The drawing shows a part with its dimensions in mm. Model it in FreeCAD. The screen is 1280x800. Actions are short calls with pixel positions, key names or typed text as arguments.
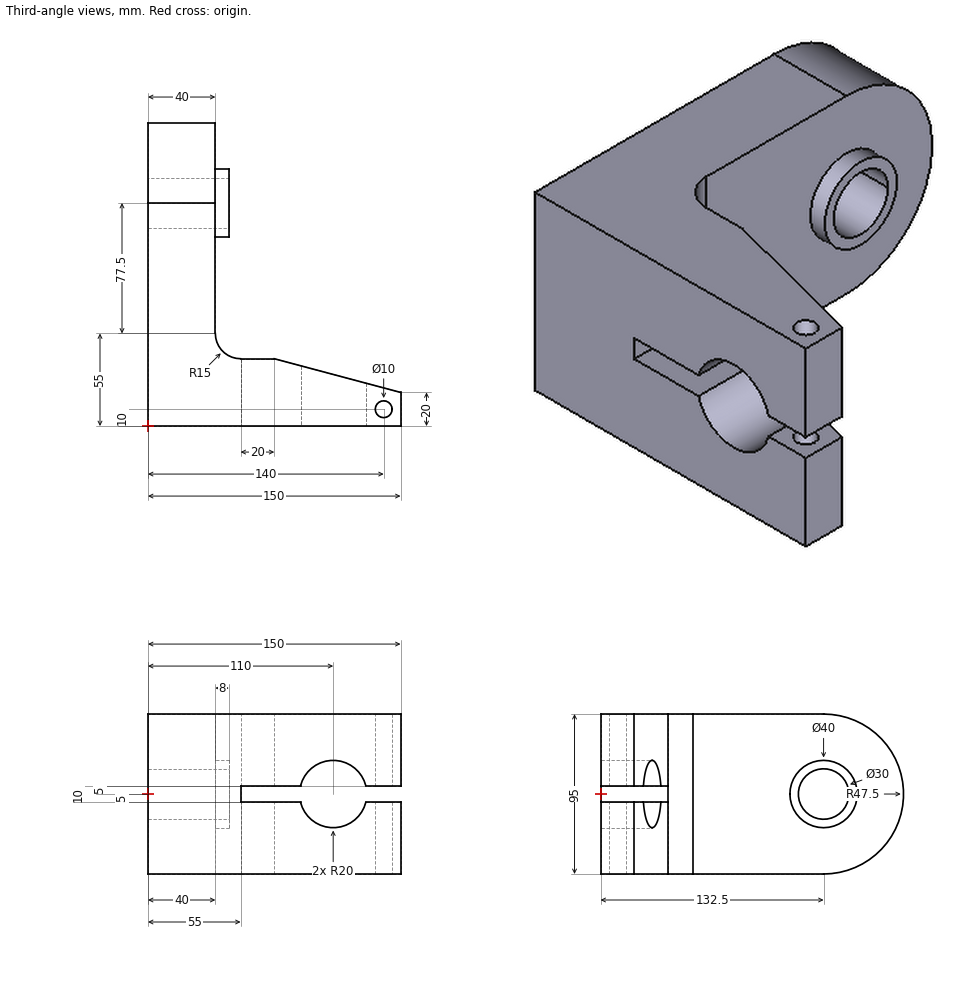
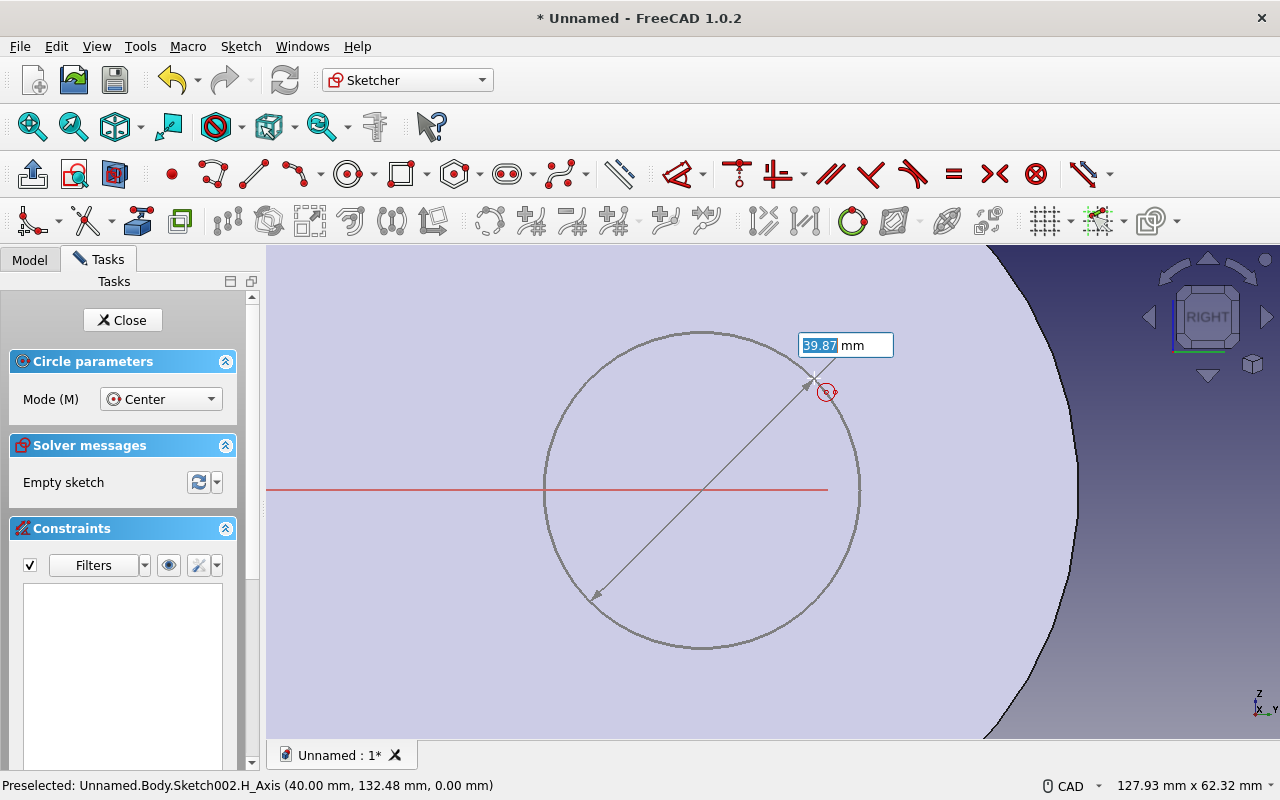
text(40)
key(Return)
key(Escape)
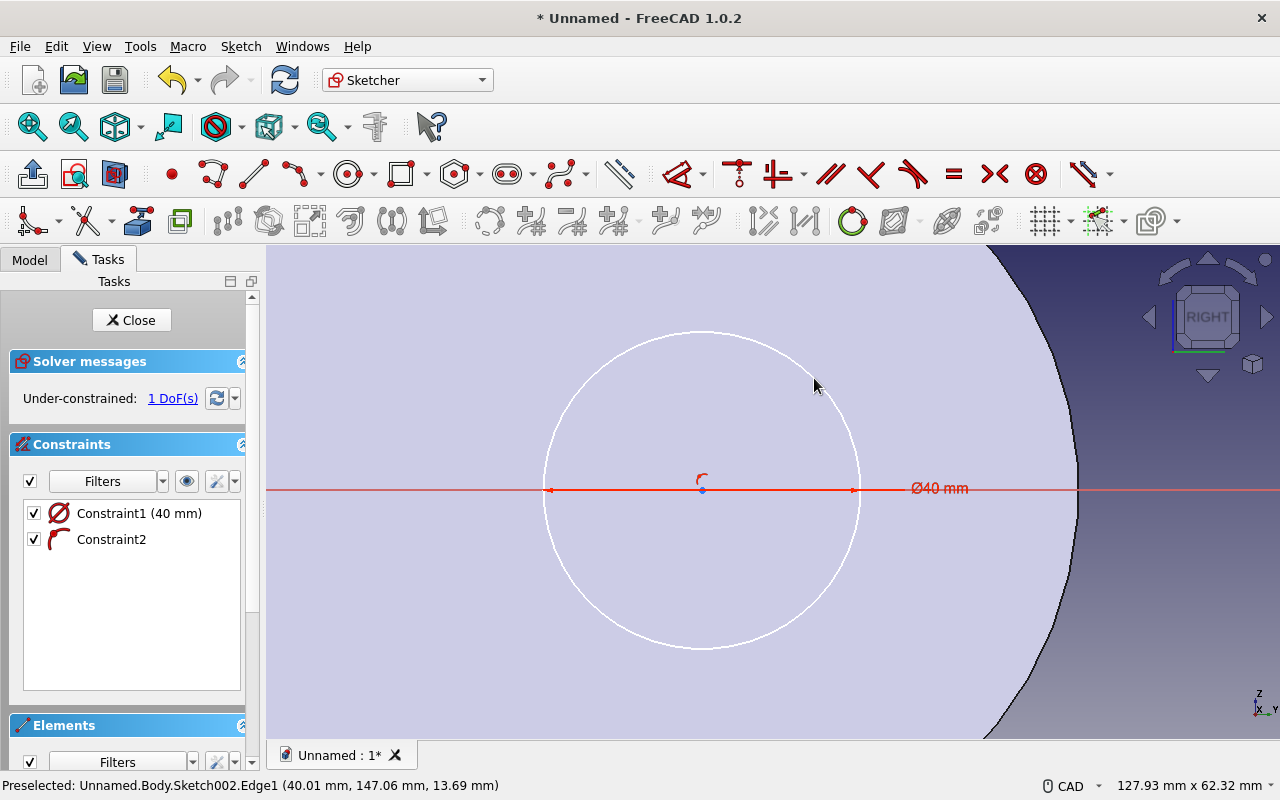
click(676, 174)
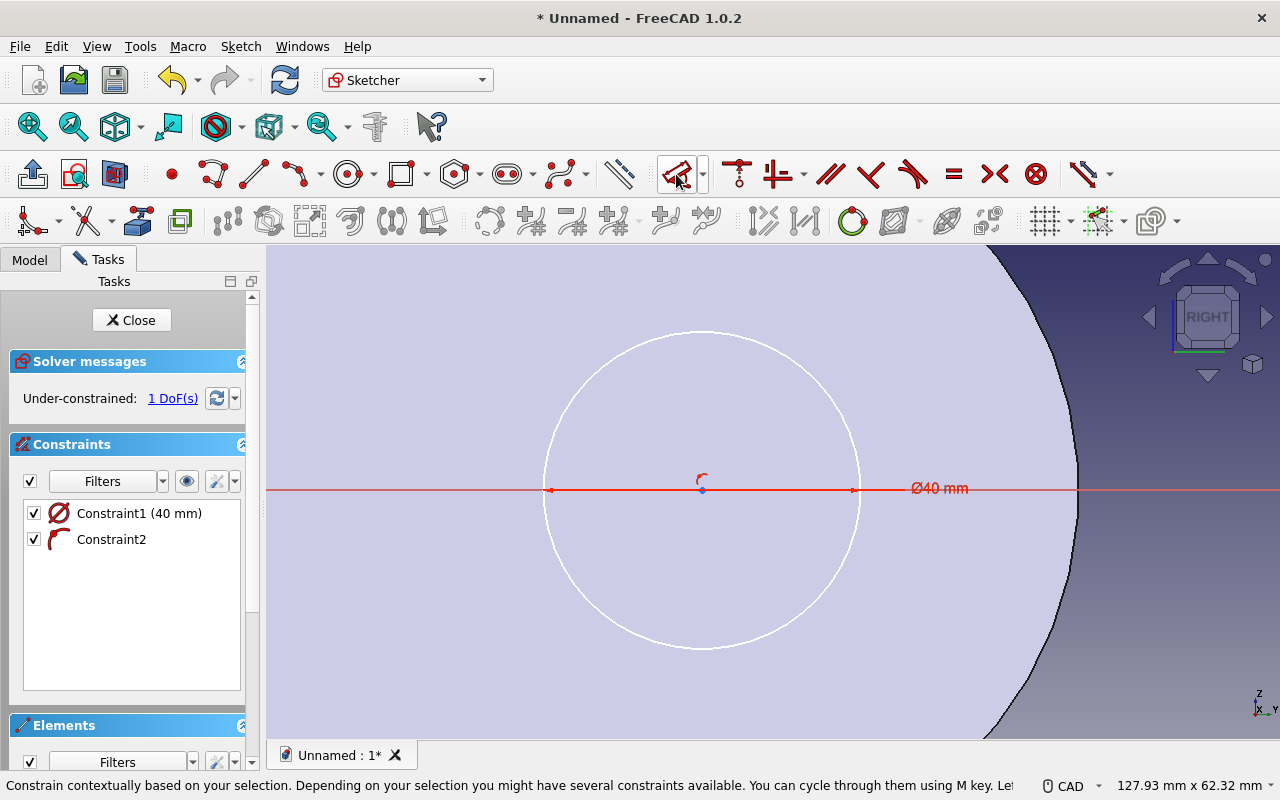
click(702, 490)
click(498, 524)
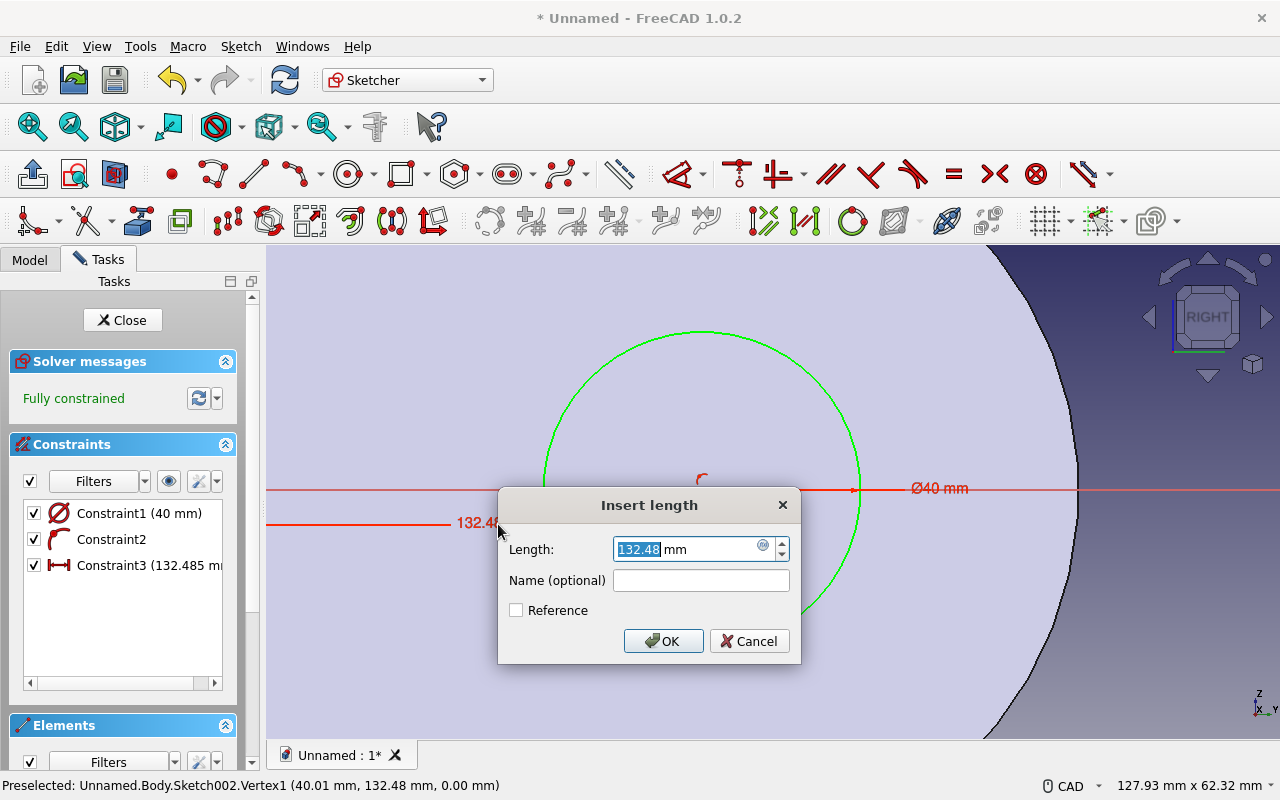
text(132.5)
key(Return)
key(Escape)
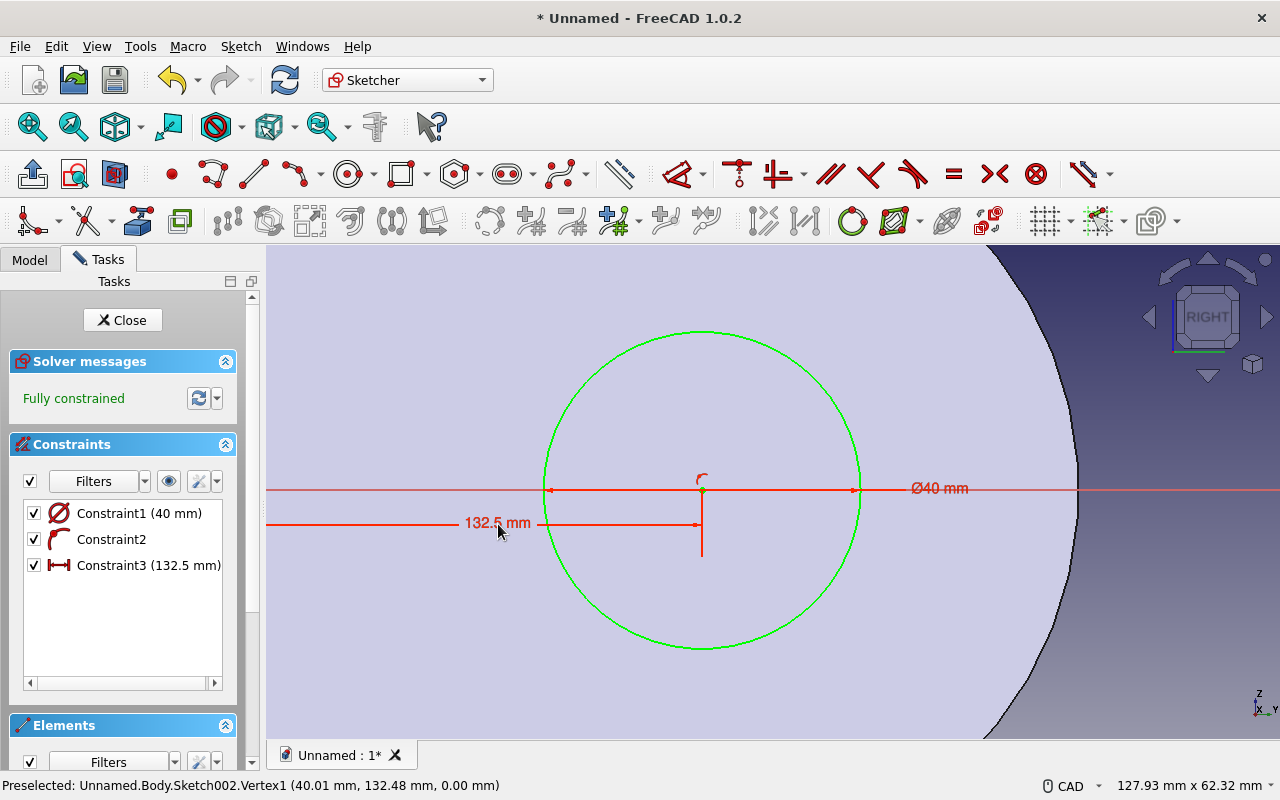
click(123, 320)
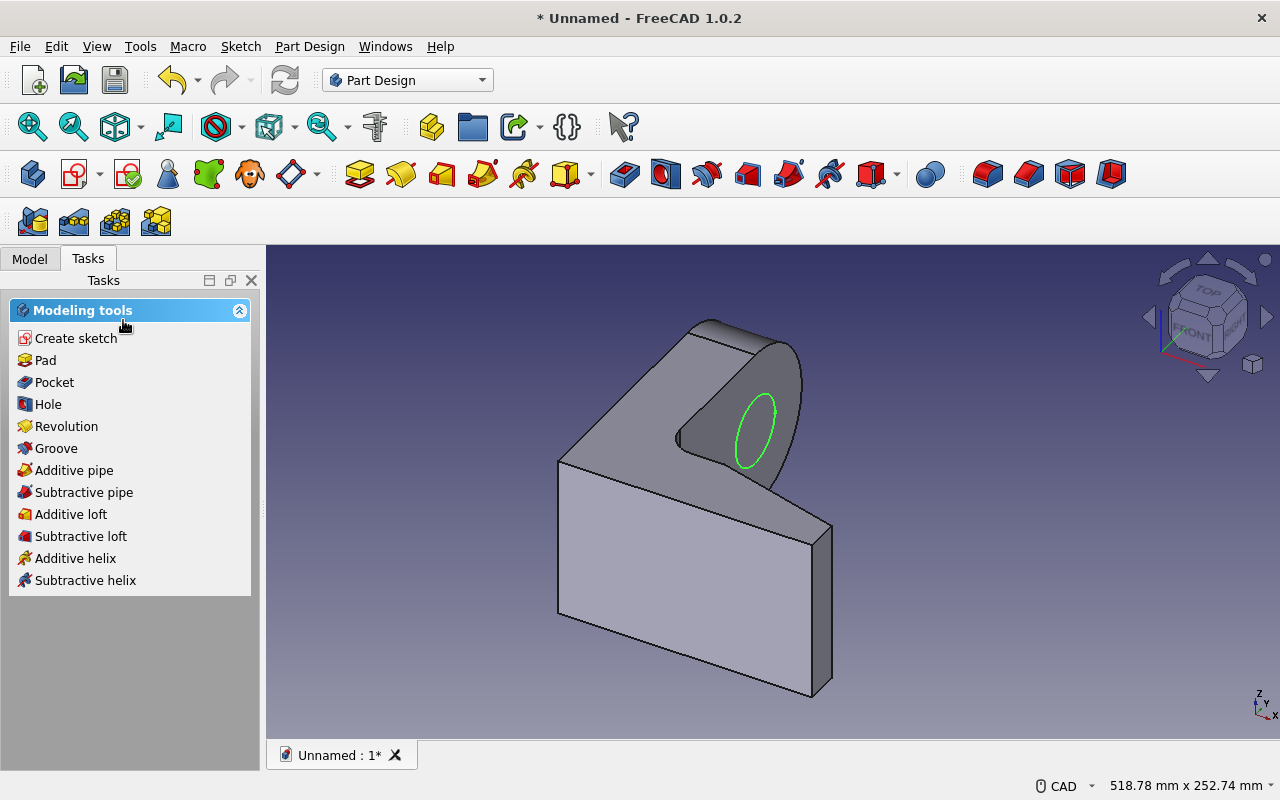
click(360, 174)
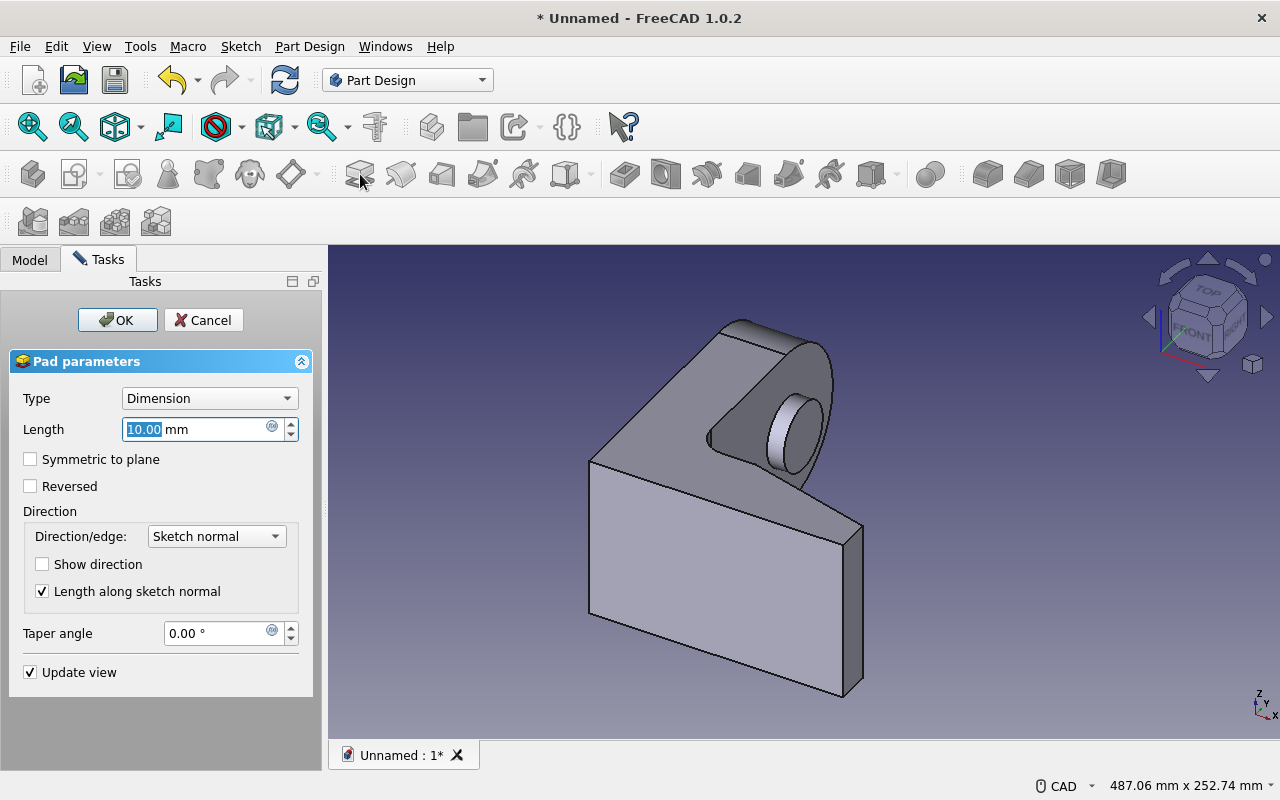
text(8)
key(Tab)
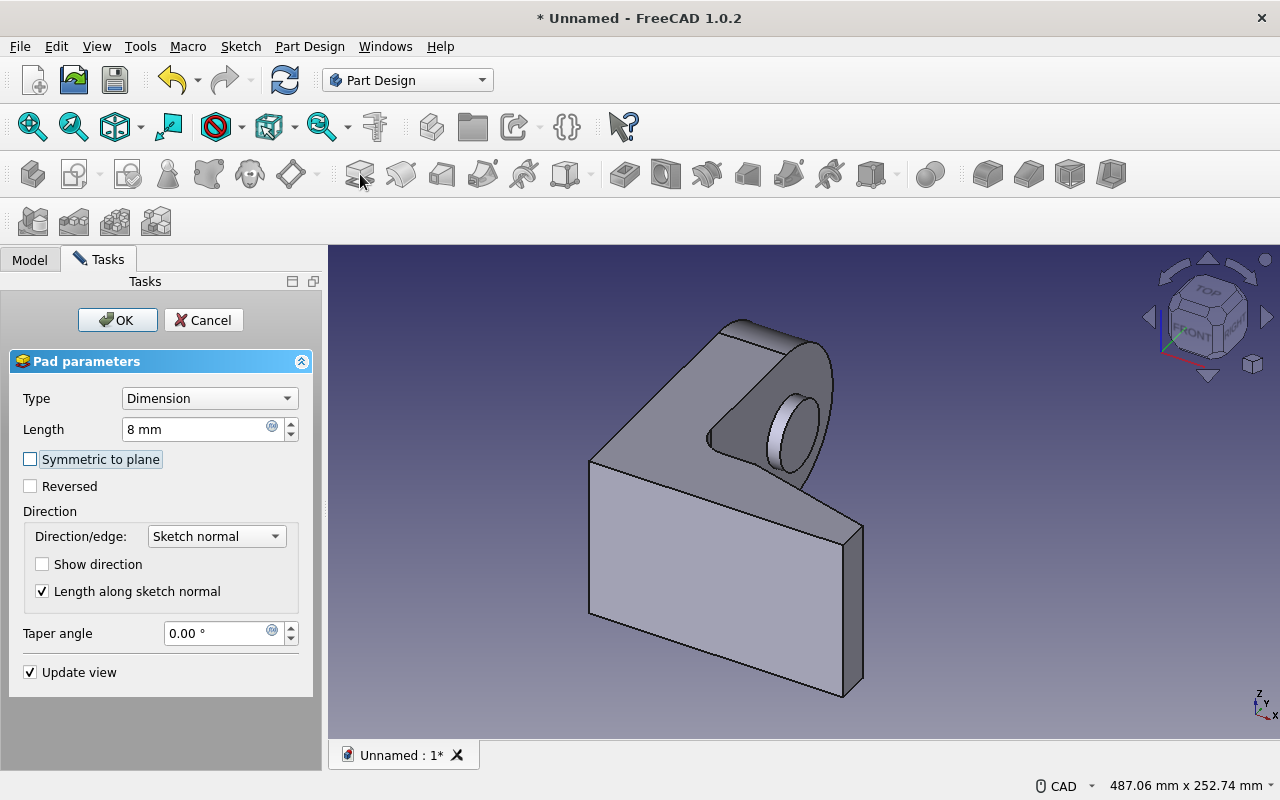
click(118, 320)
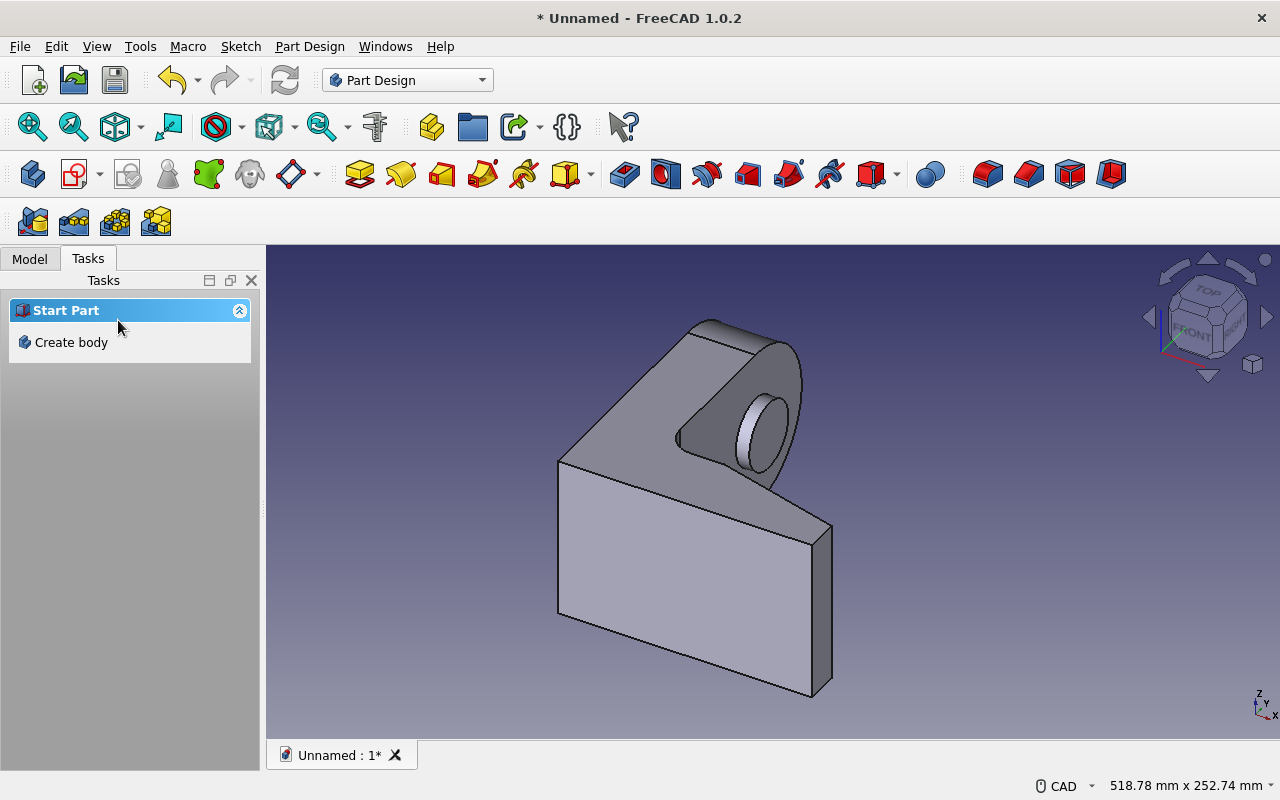
click(769, 435)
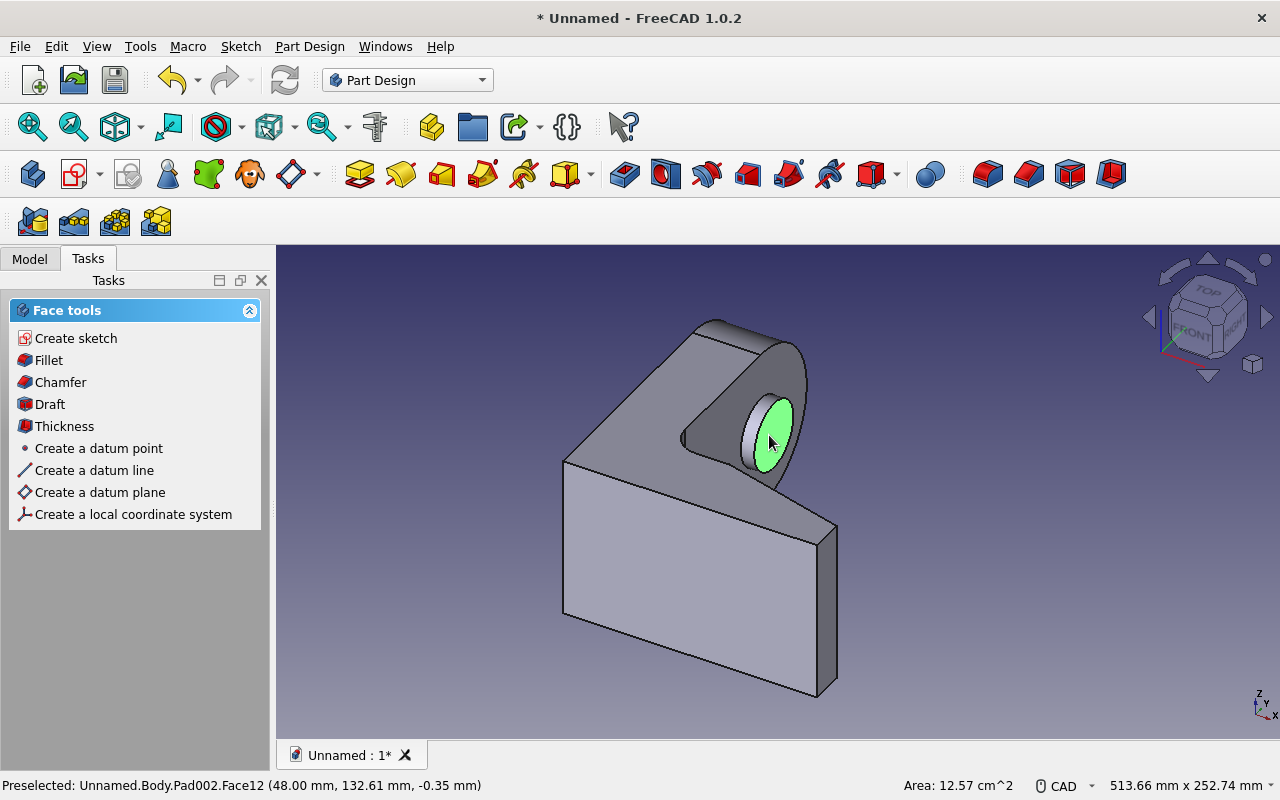
click(74, 174)